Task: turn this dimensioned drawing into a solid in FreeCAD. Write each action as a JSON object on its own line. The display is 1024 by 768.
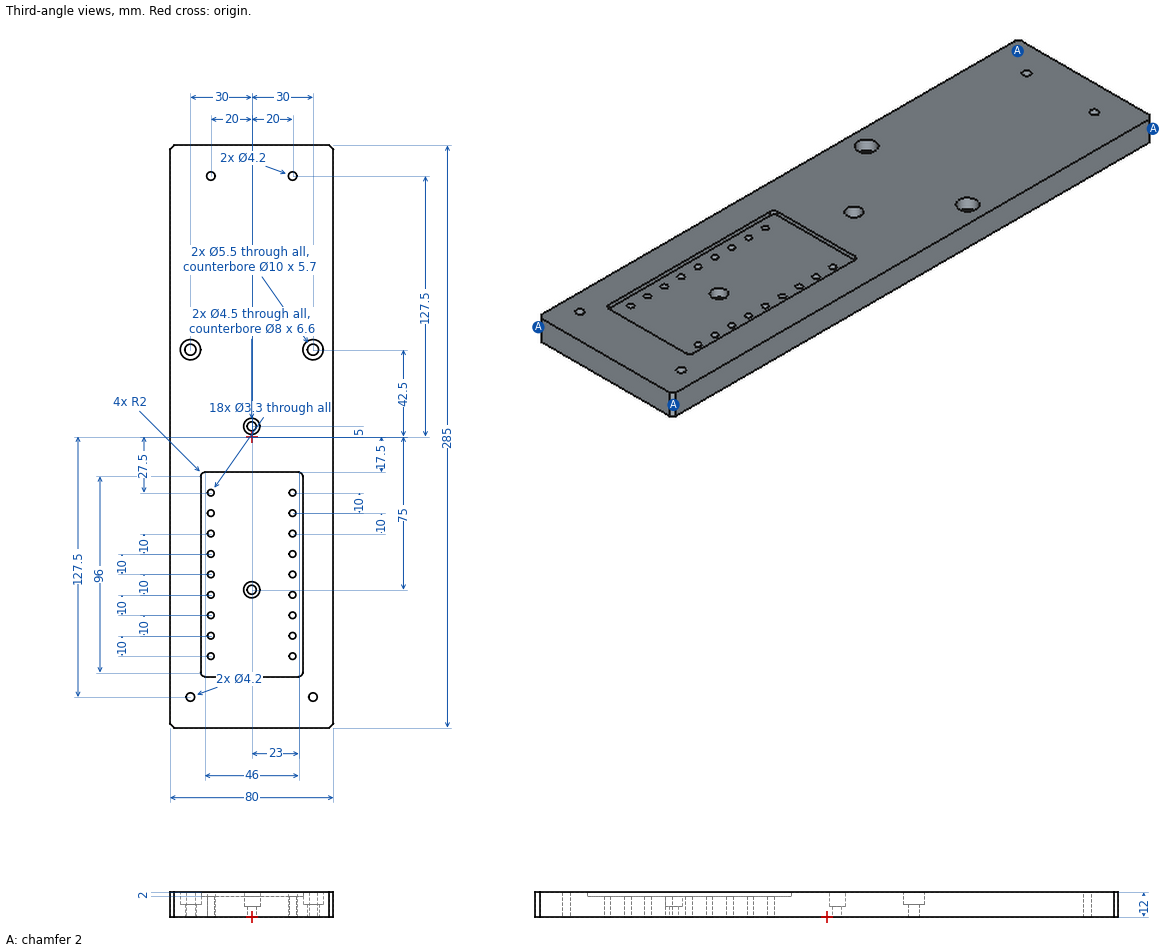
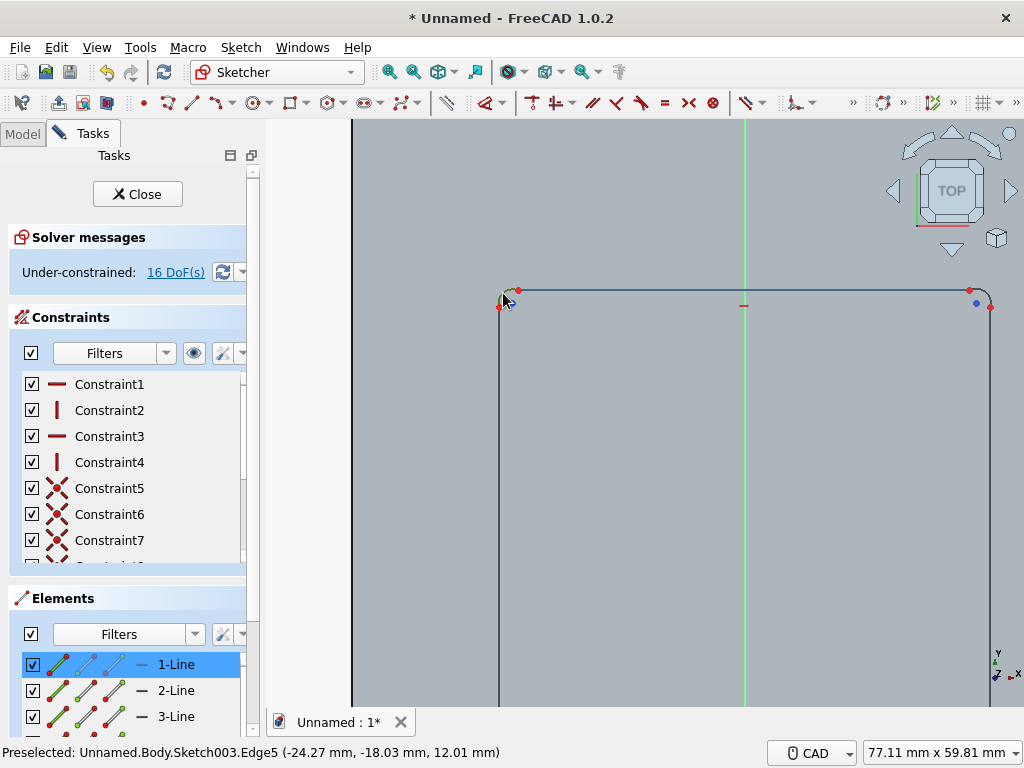
{"action": "key", "text": "t"}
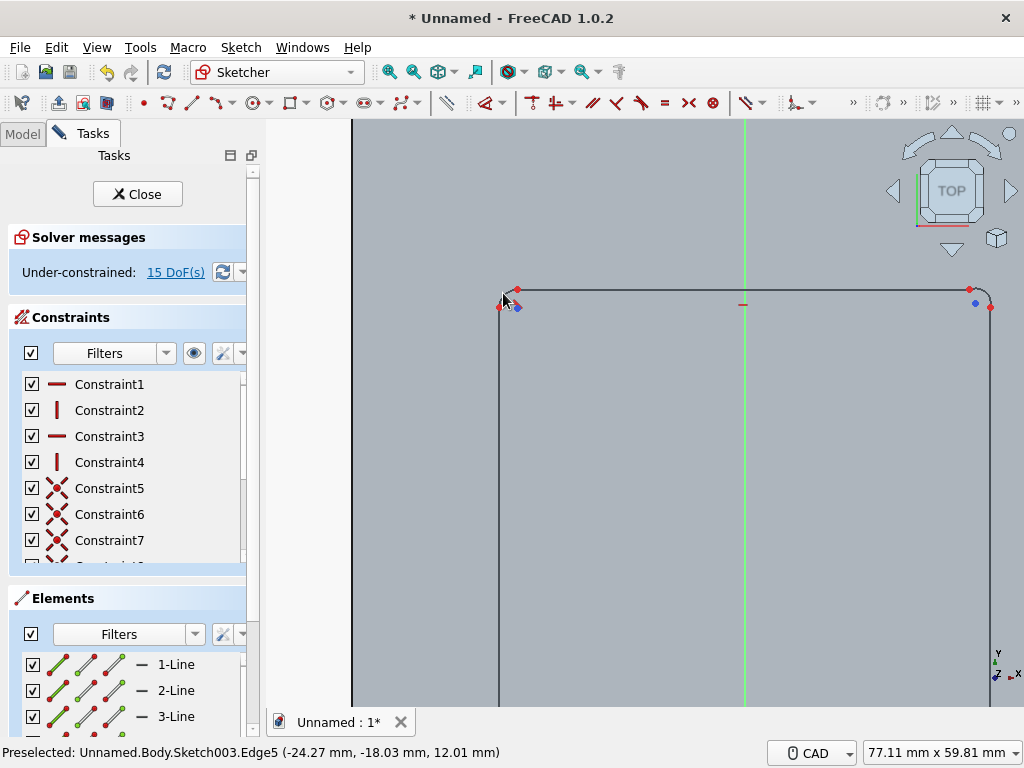
{"action": "left_click", "coordinate": [834, 290]}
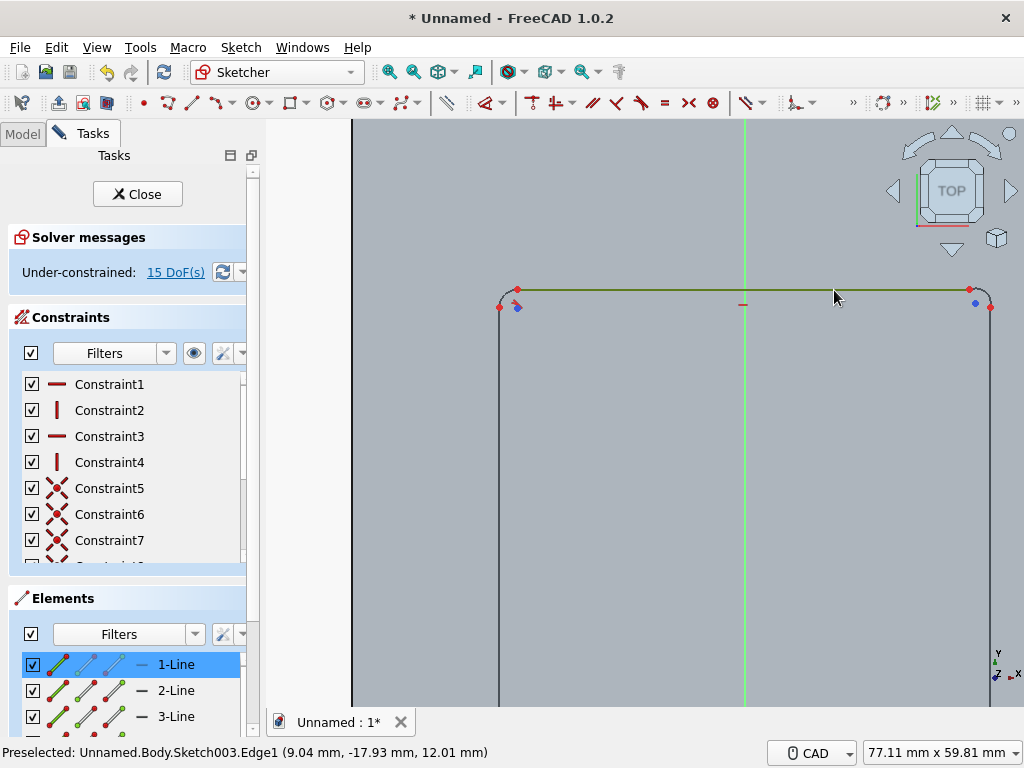
{"action": "scroll", "coordinate": [504, 293], "scroll_direction": "down", "scroll_amount": 6}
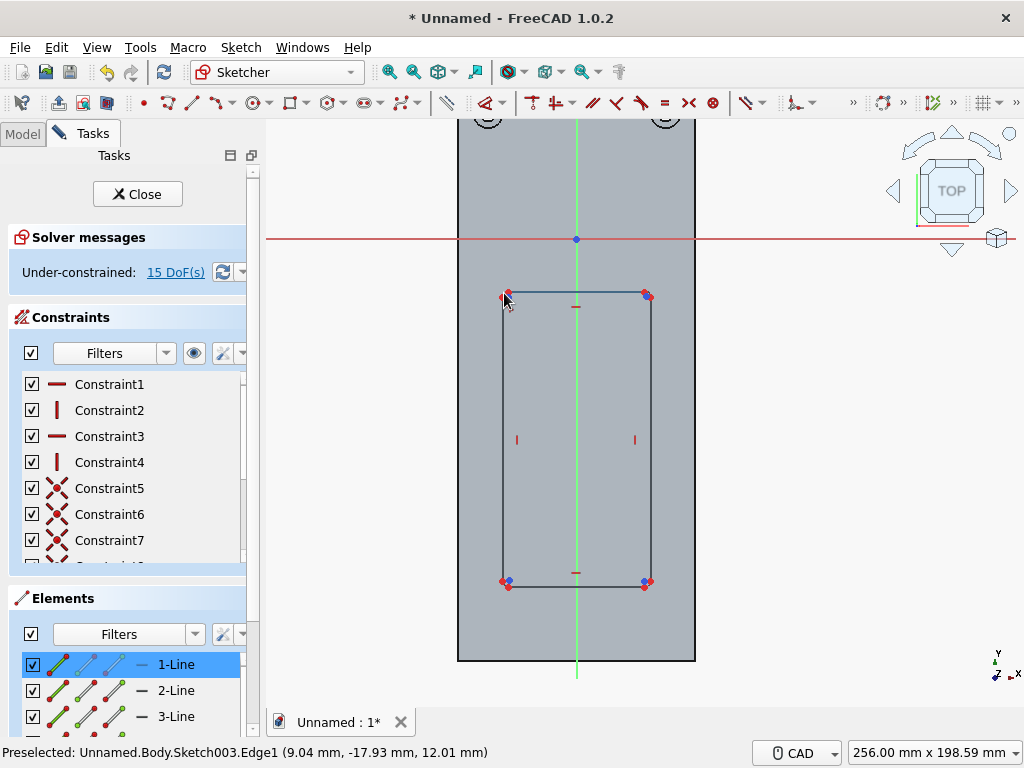
{"action": "scroll", "coordinate": [650, 295], "scroll_direction": "up", "scroll_amount": 8}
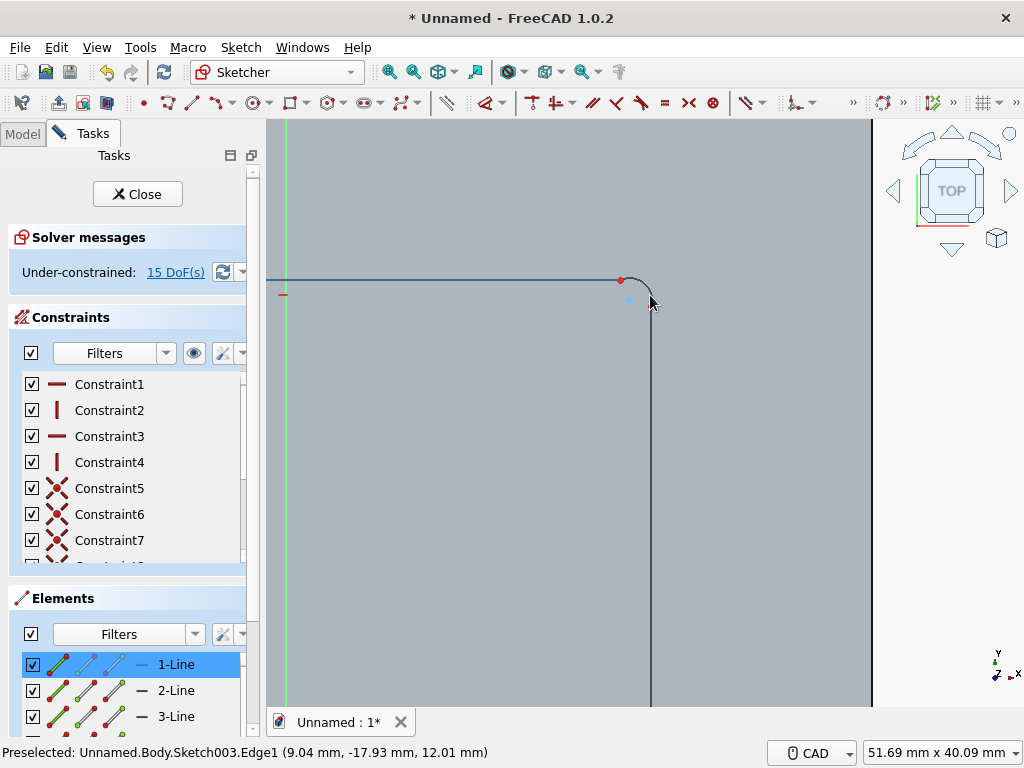
{"action": "left_click", "coordinate": [650, 292]}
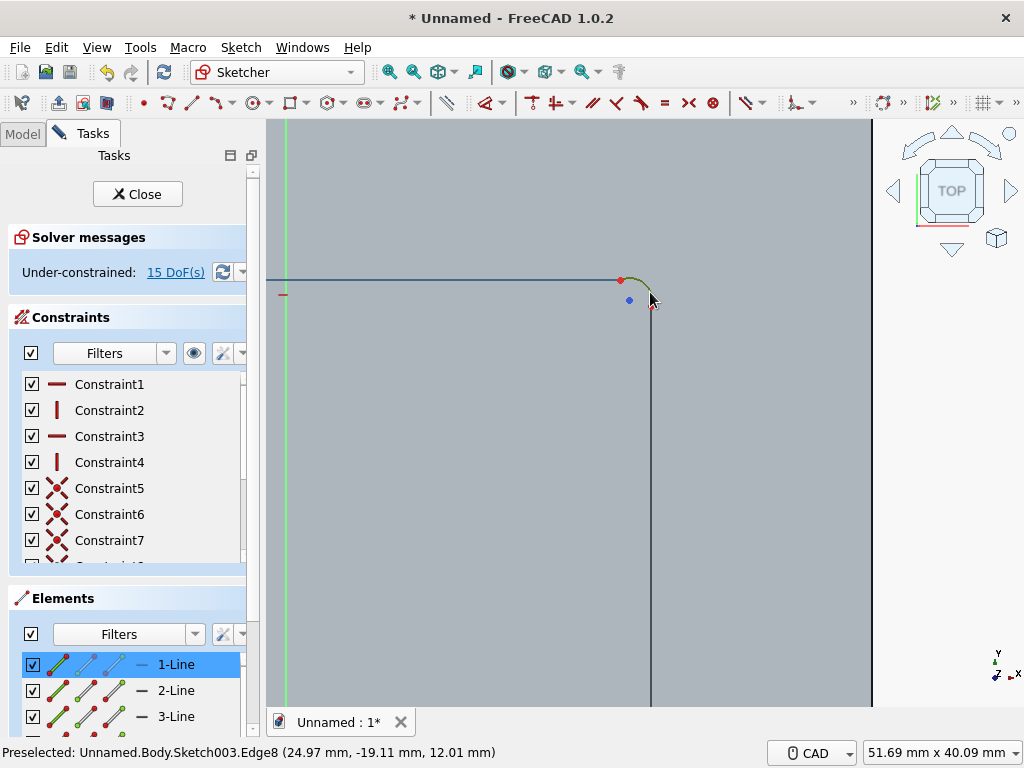
{"action": "key", "text": "t"}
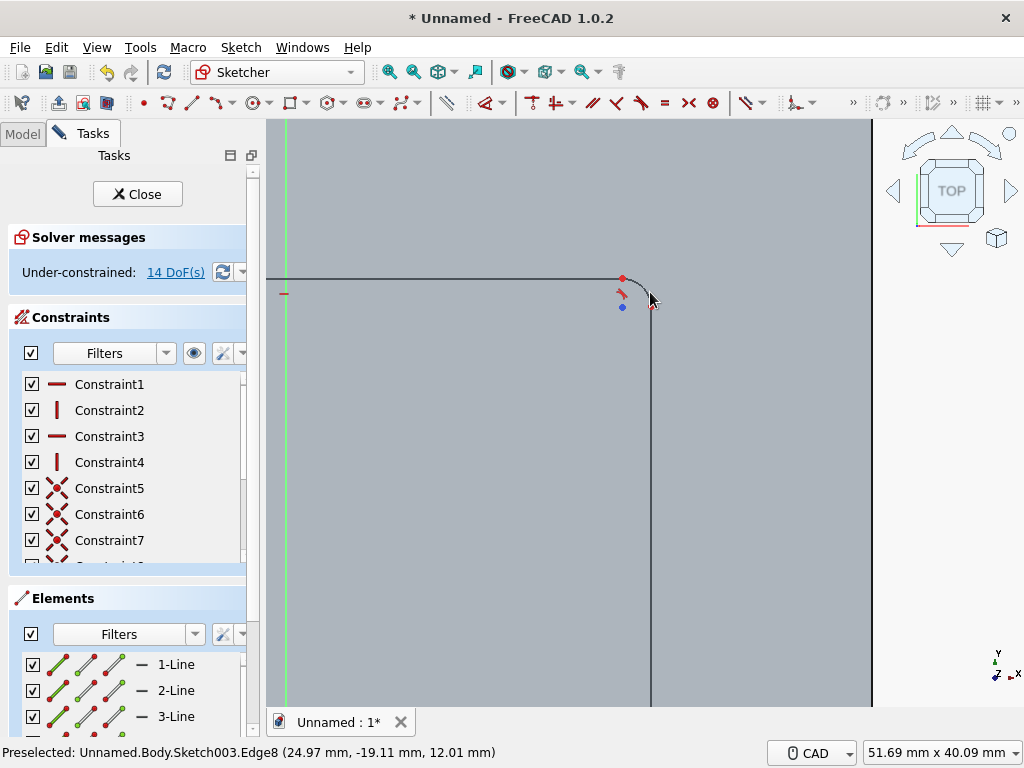
{"action": "scroll", "coordinate": [650, 295], "scroll_direction": "down", "scroll_amount": 8}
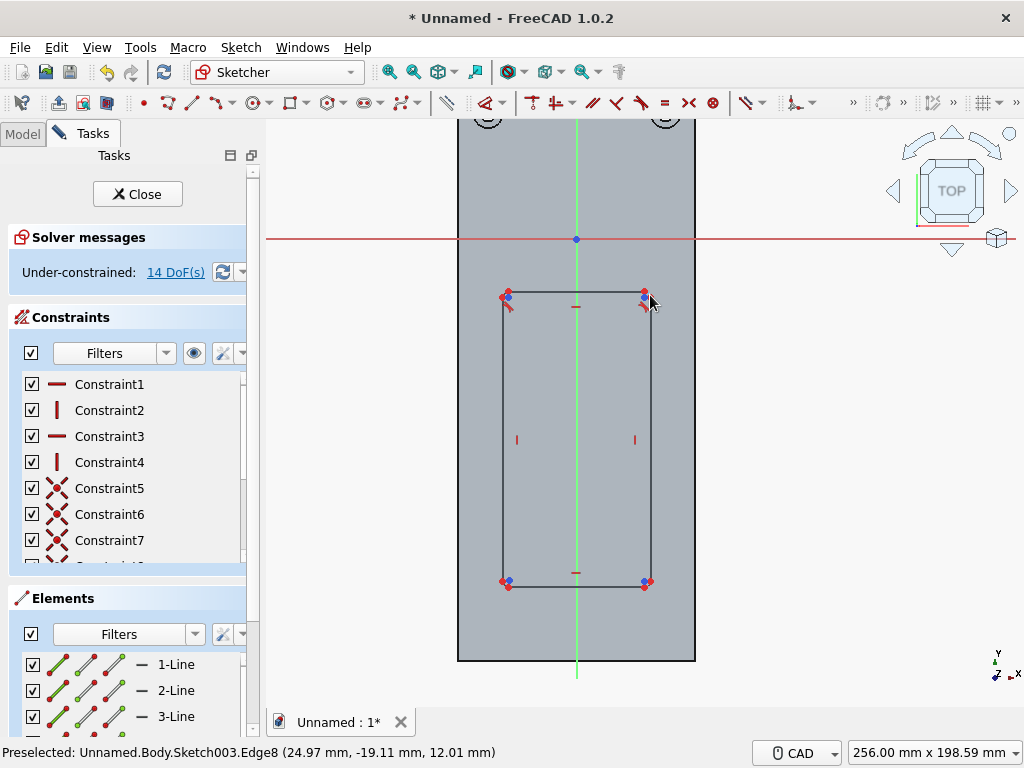
{"action": "left_click", "coordinate": [503, 383]}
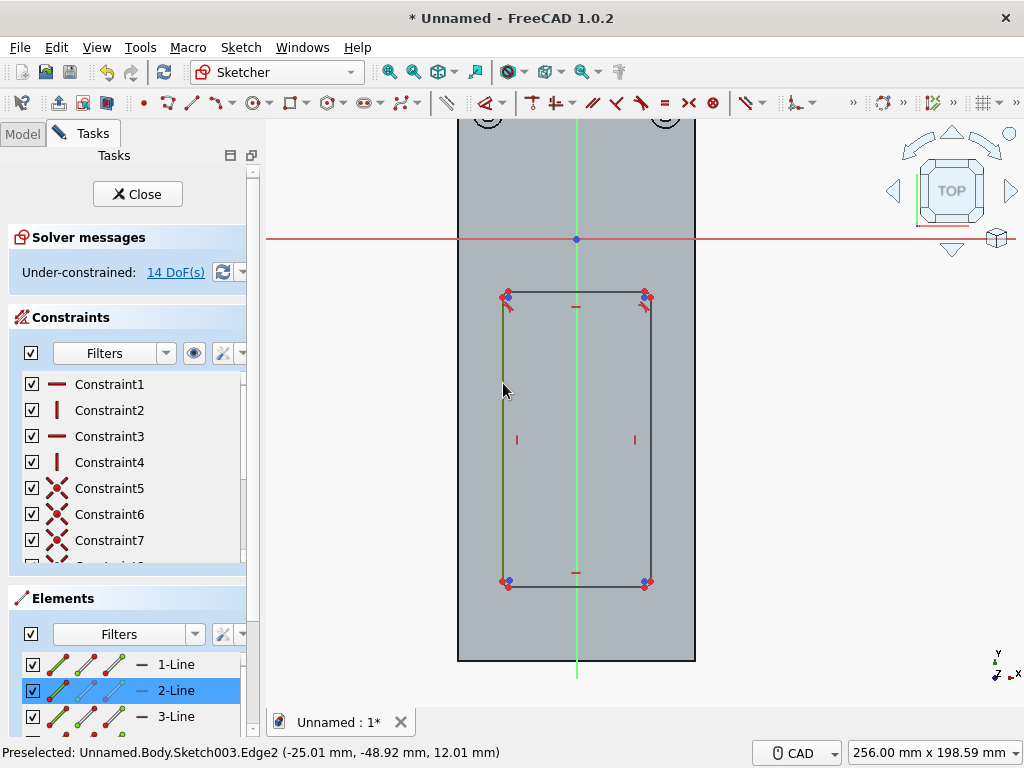
{"action": "scroll", "coordinate": [505, 294], "scroll_direction": "up", "scroll_amount": 6}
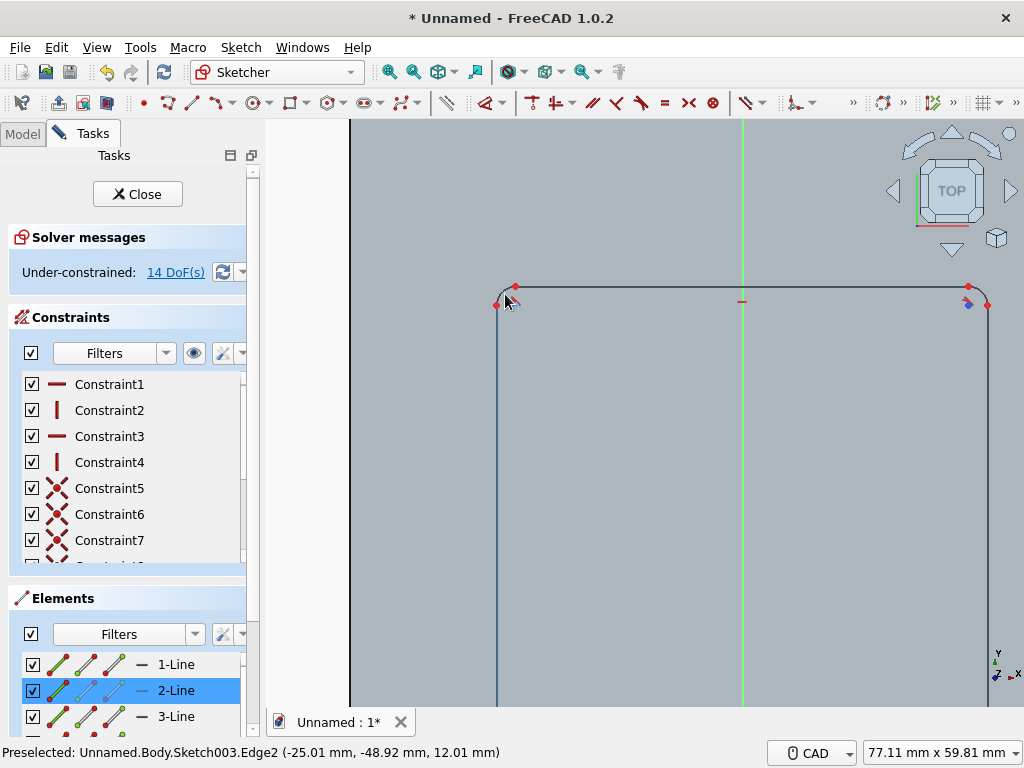
{"action": "left_click", "coordinate": [503, 292]}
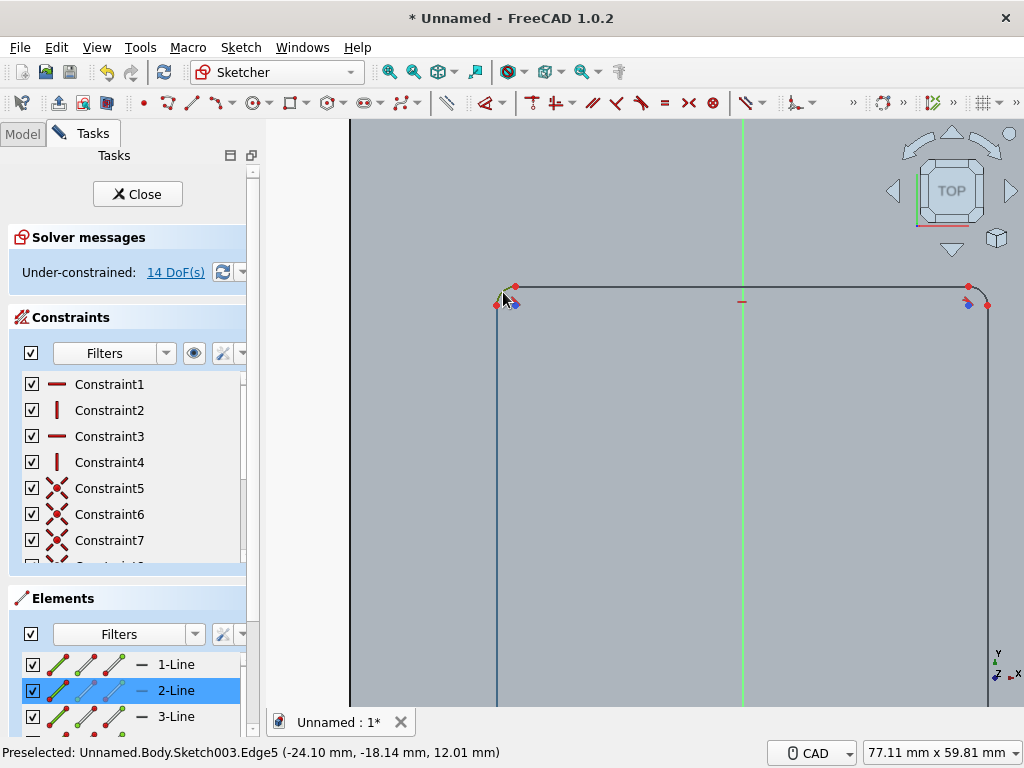
{"action": "key", "text": "t"}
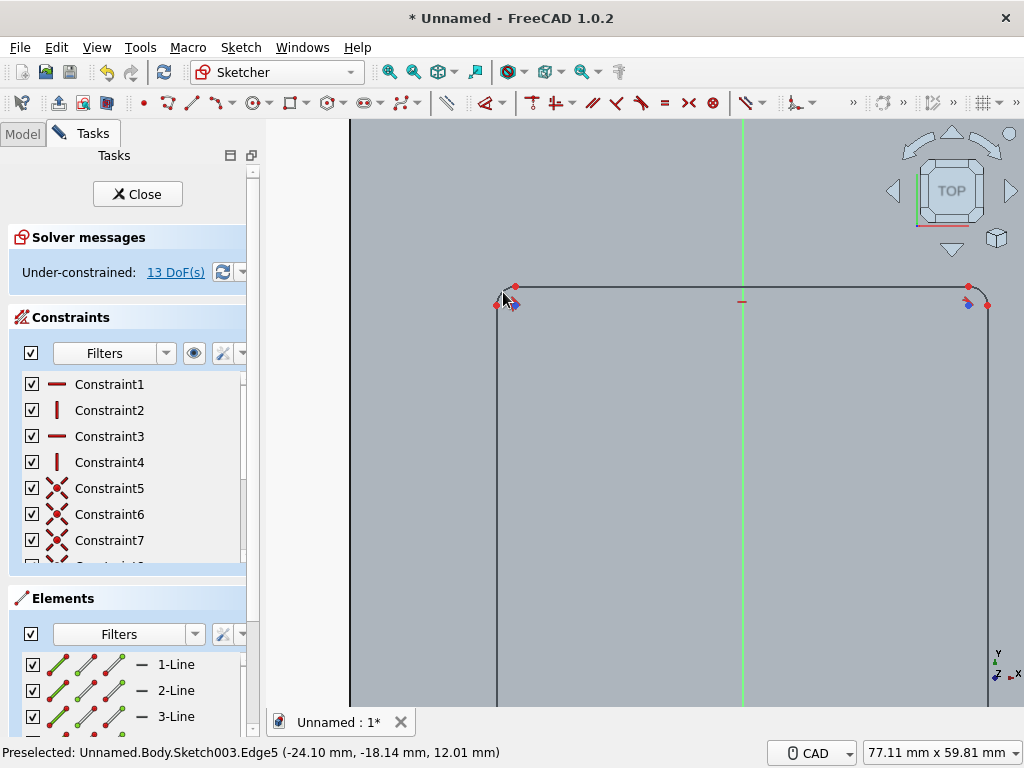
{"action": "left_click", "coordinate": [497, 589]}